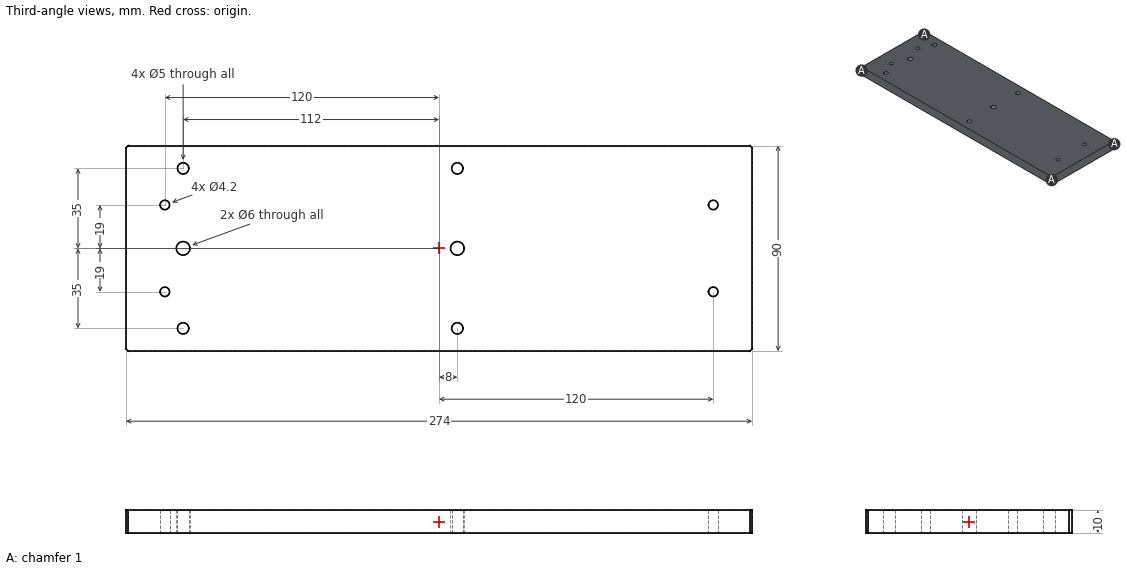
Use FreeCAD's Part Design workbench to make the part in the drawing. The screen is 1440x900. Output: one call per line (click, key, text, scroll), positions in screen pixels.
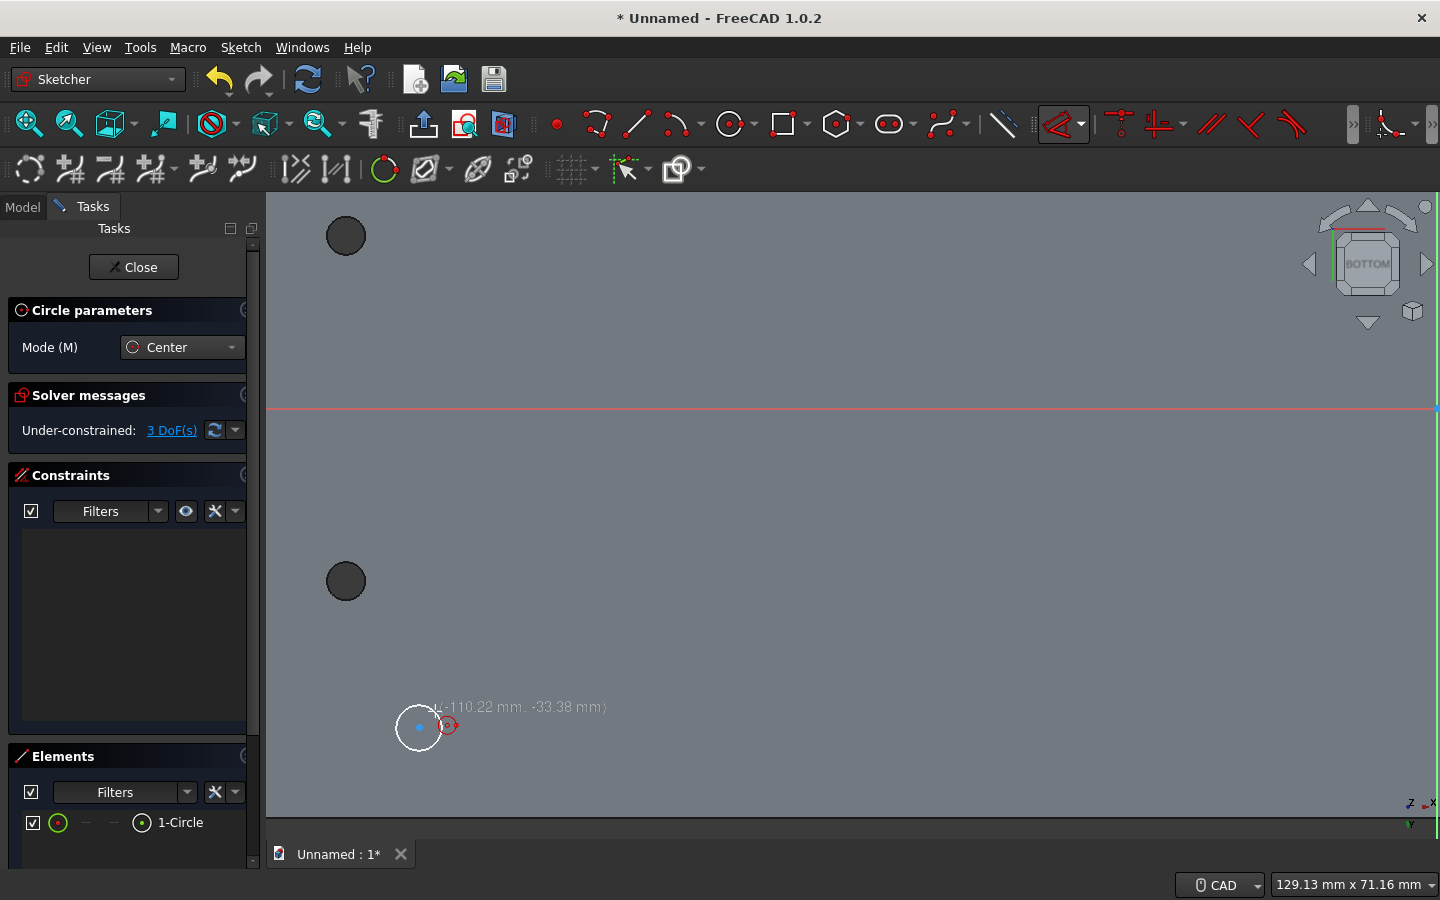
scroll(419, 733, down, 2)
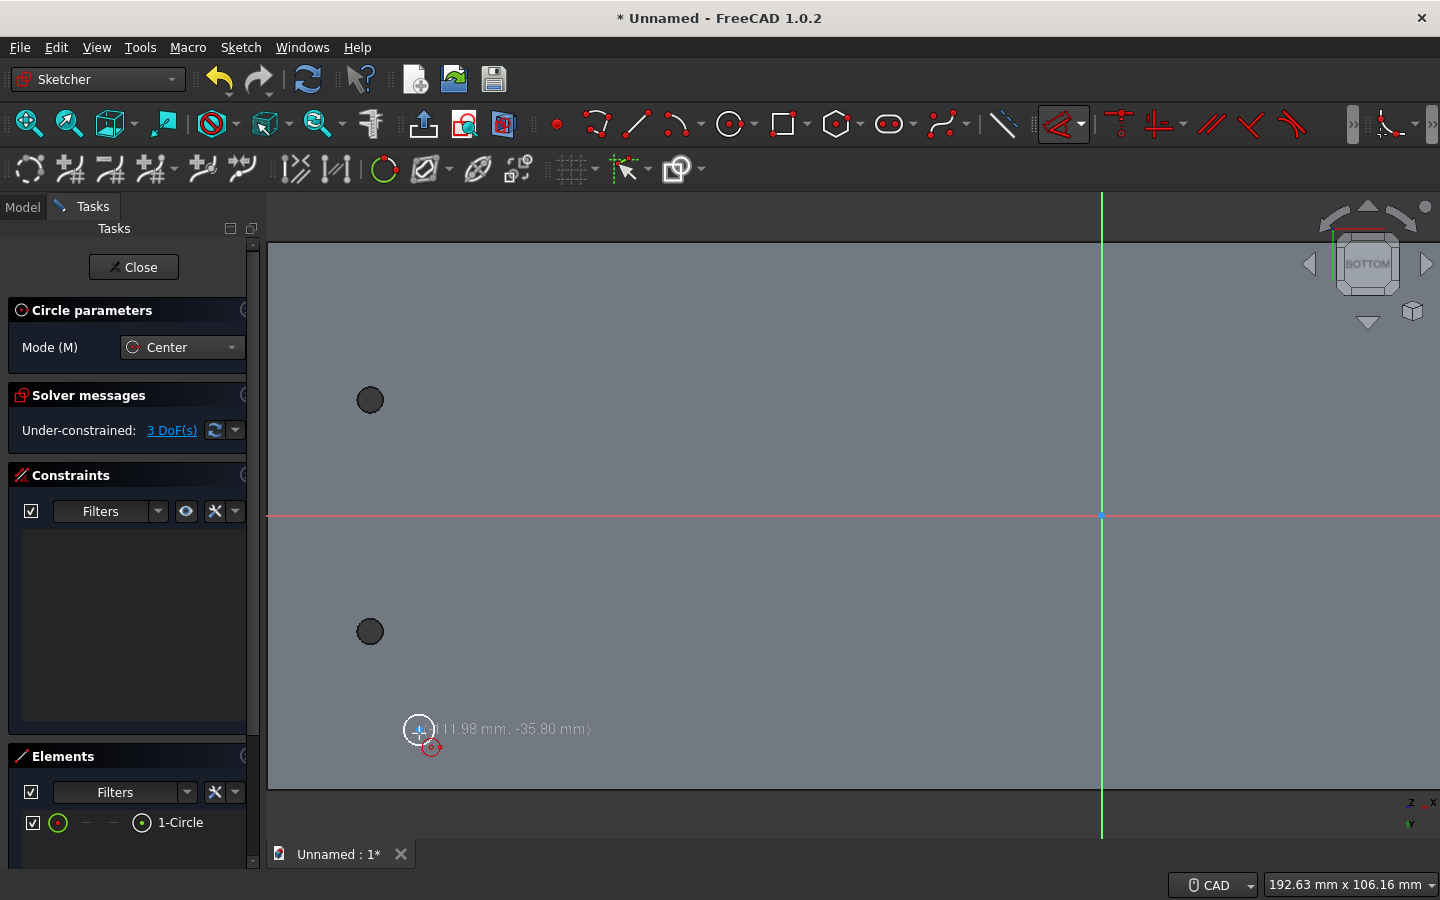
scroll(419, 302, up, 2)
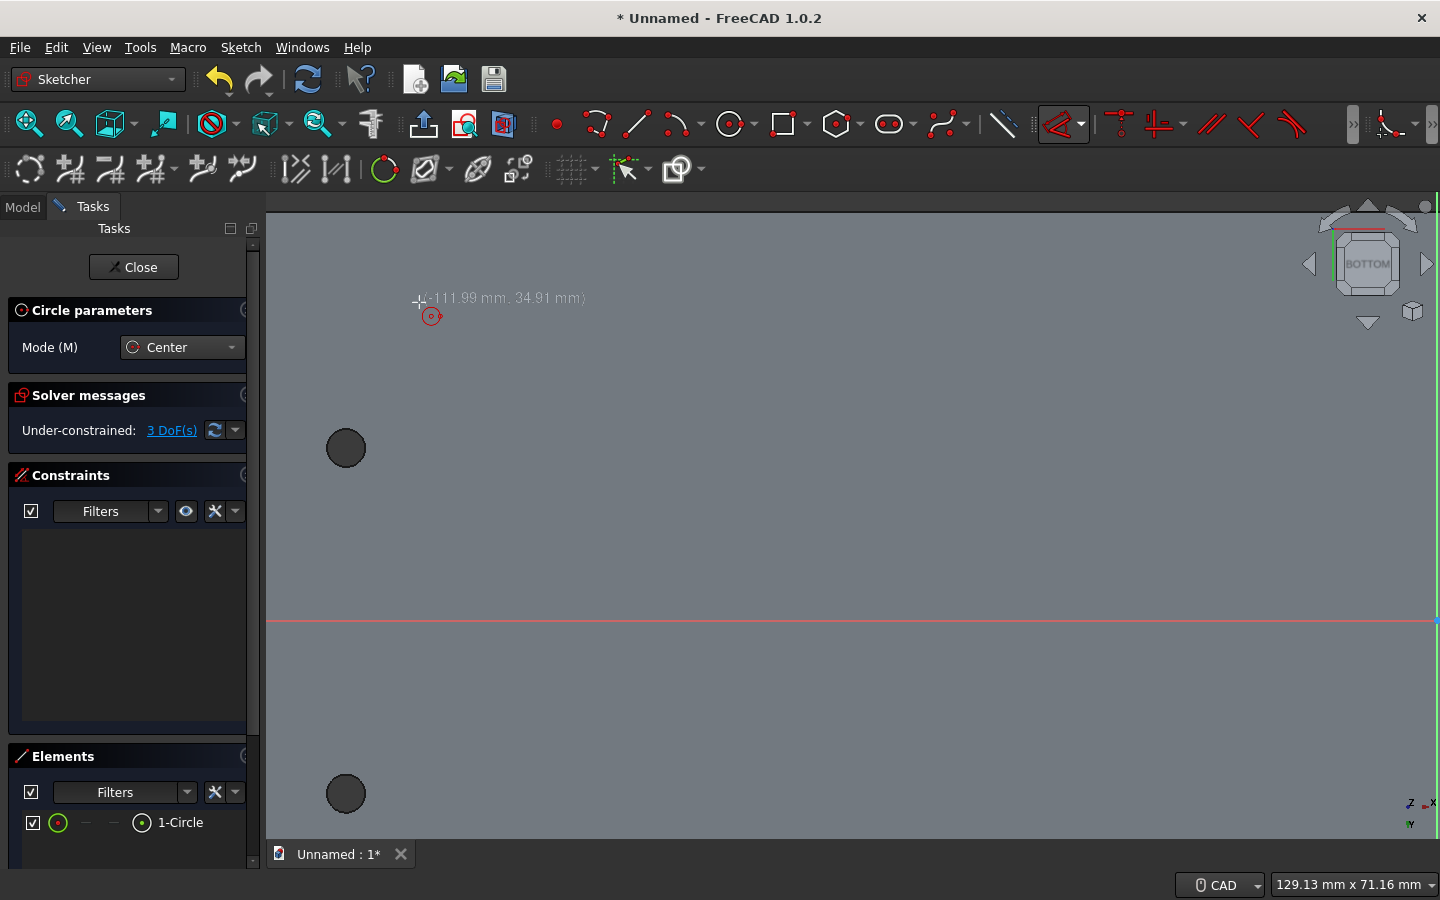
click(419, 303)
click(435, 287)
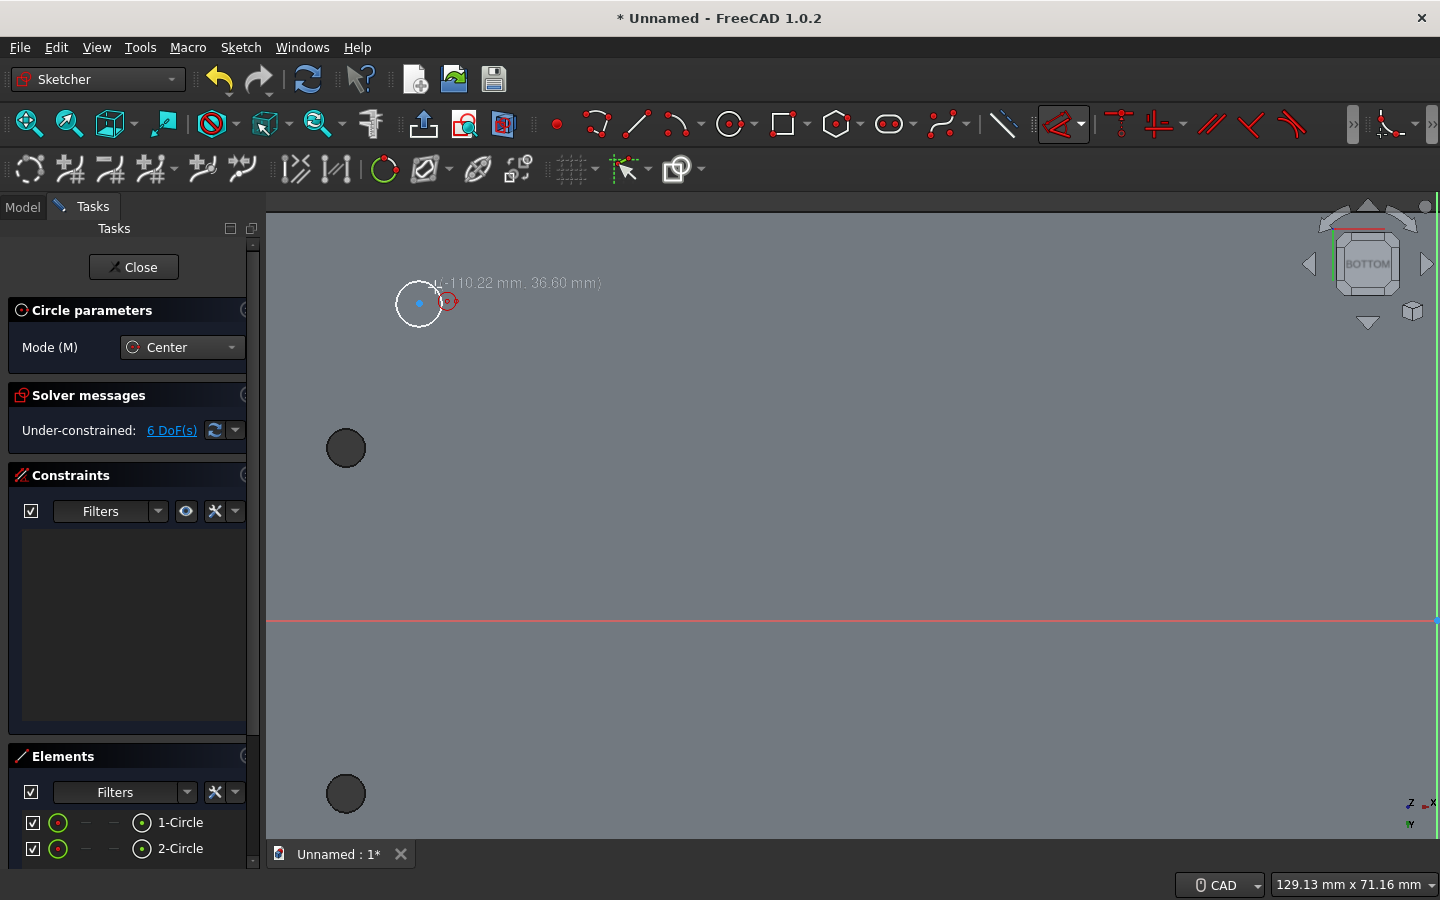
scroll(419, 301, down, 2)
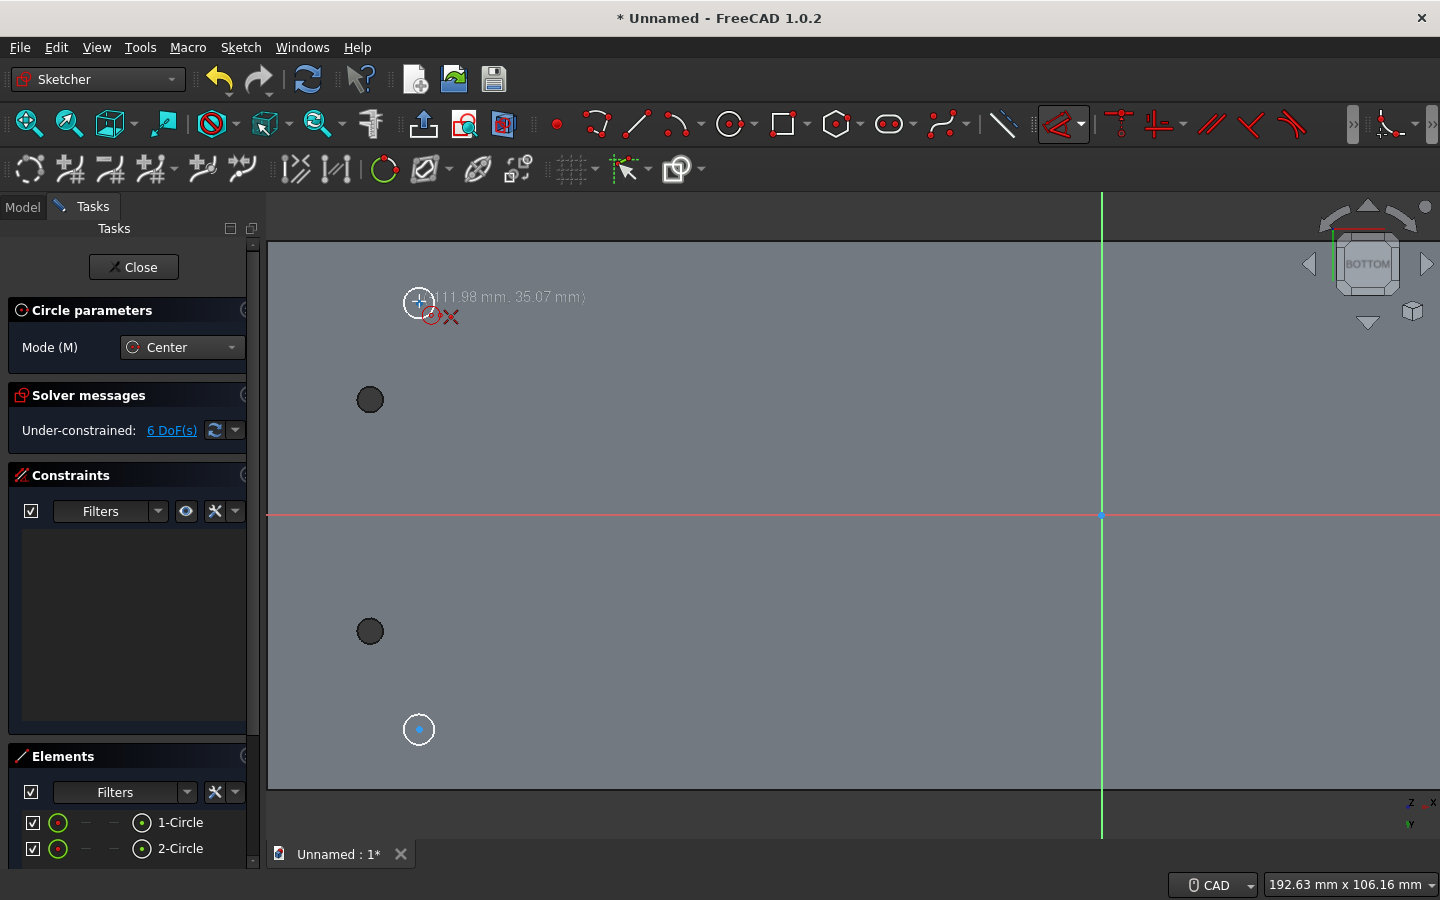
scroll(1150, 302, up, 2)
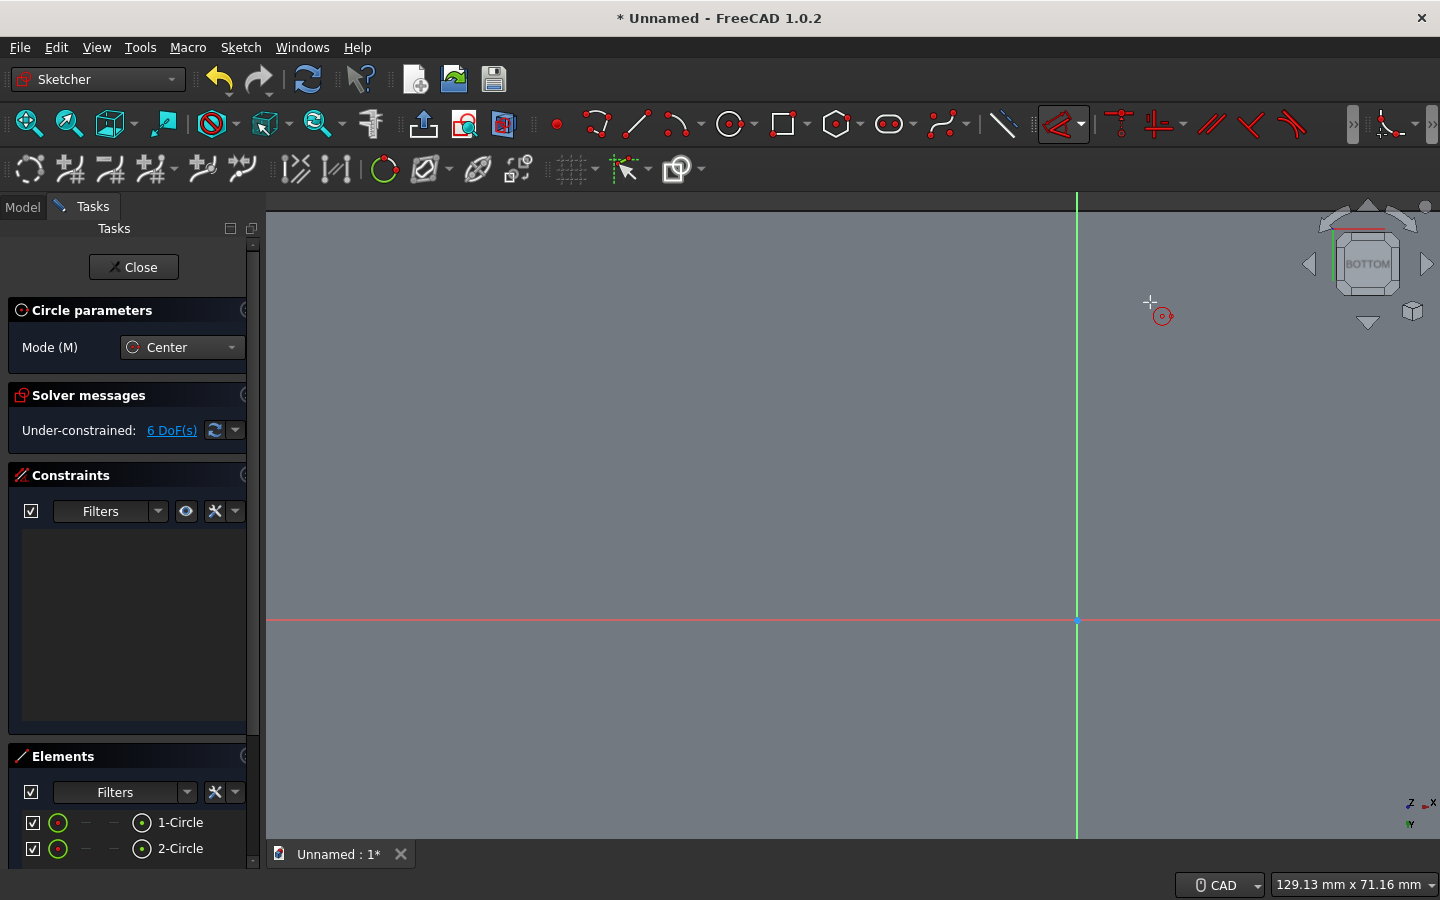
click(1150, 302)
click(1166, 286)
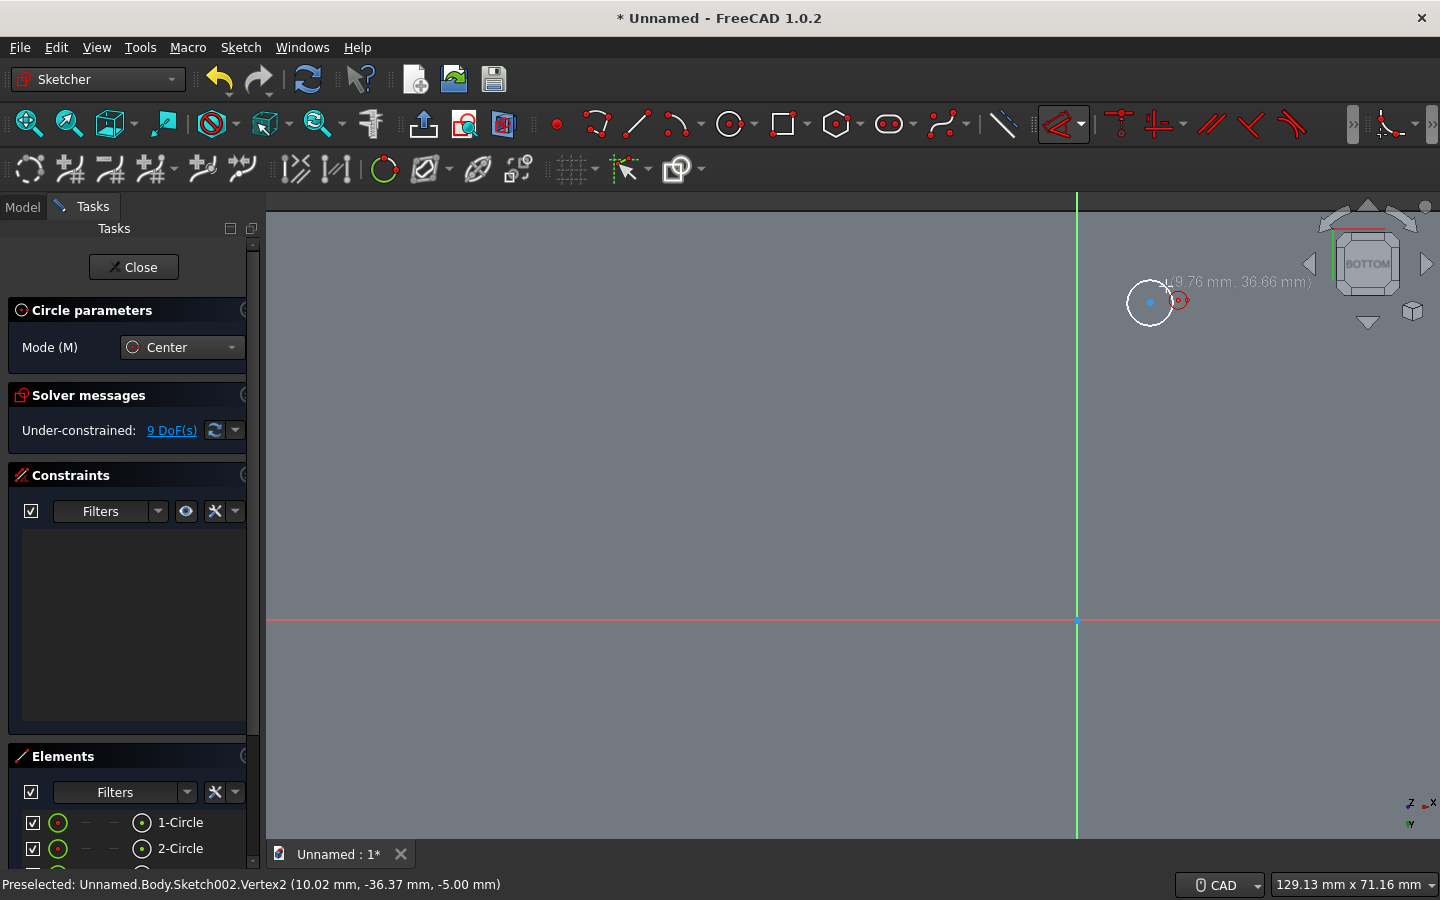
scroll(1150, 302, down, 2)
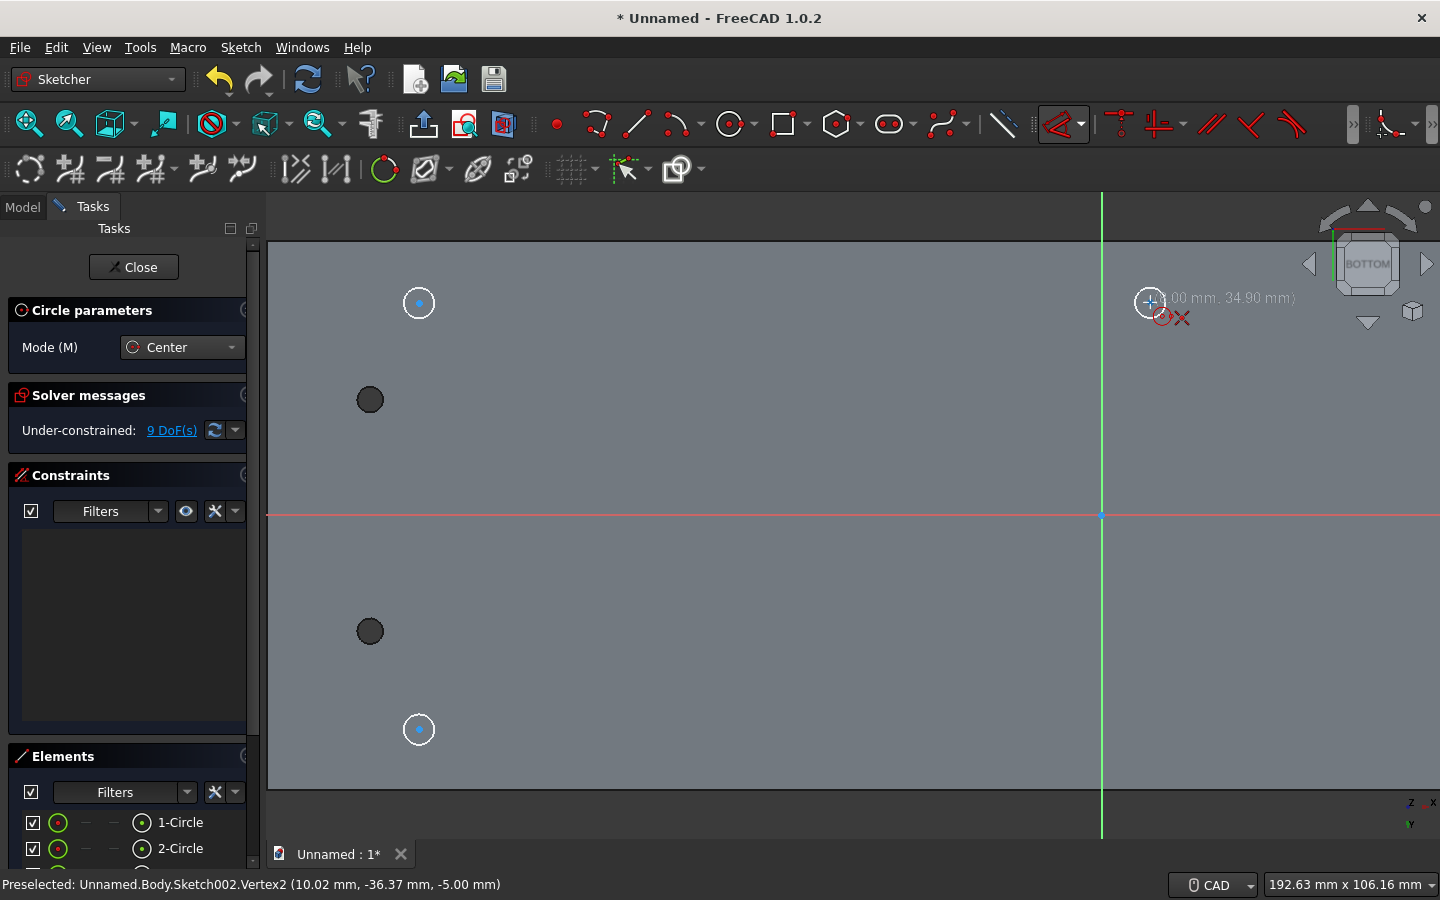
scroll(1150, 729, up, 2)